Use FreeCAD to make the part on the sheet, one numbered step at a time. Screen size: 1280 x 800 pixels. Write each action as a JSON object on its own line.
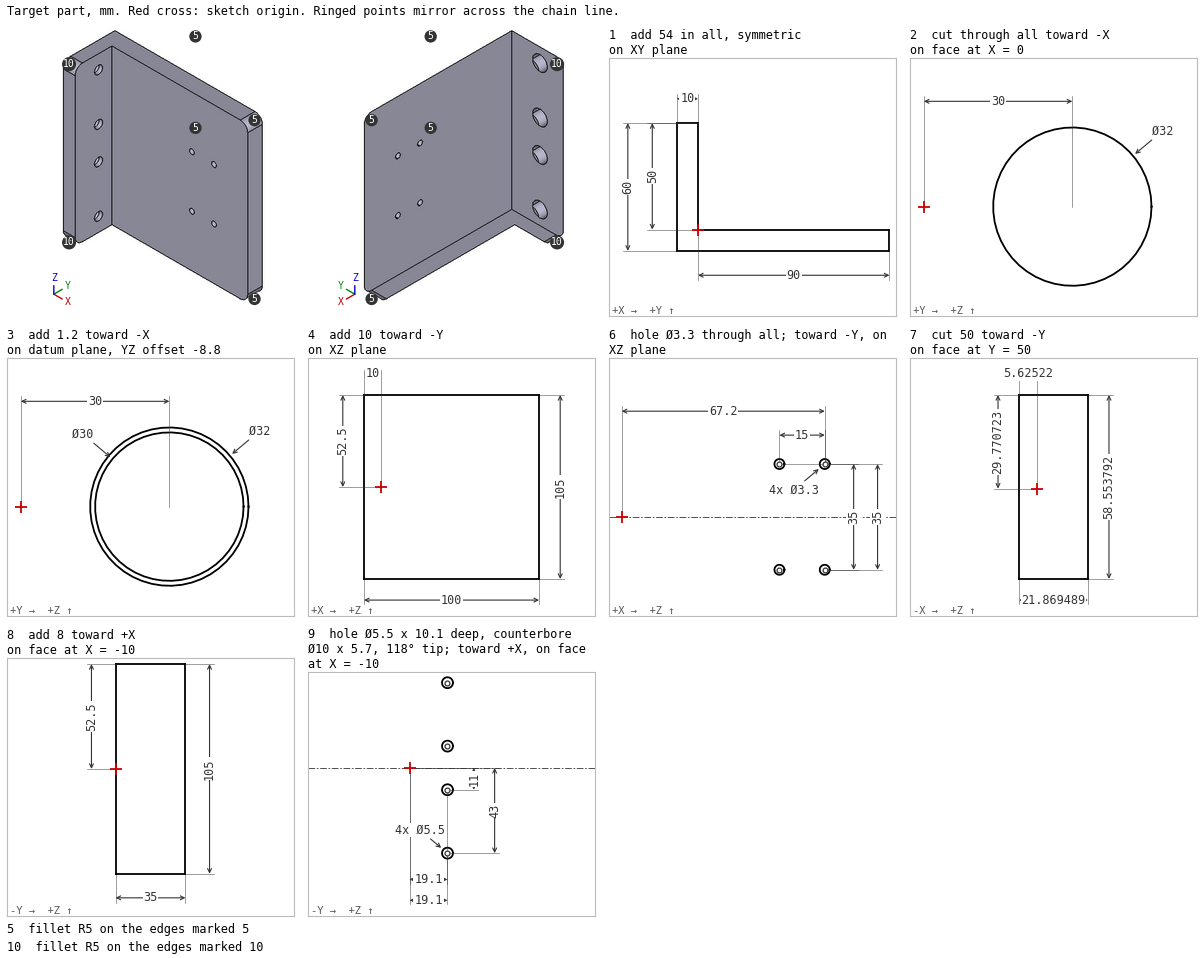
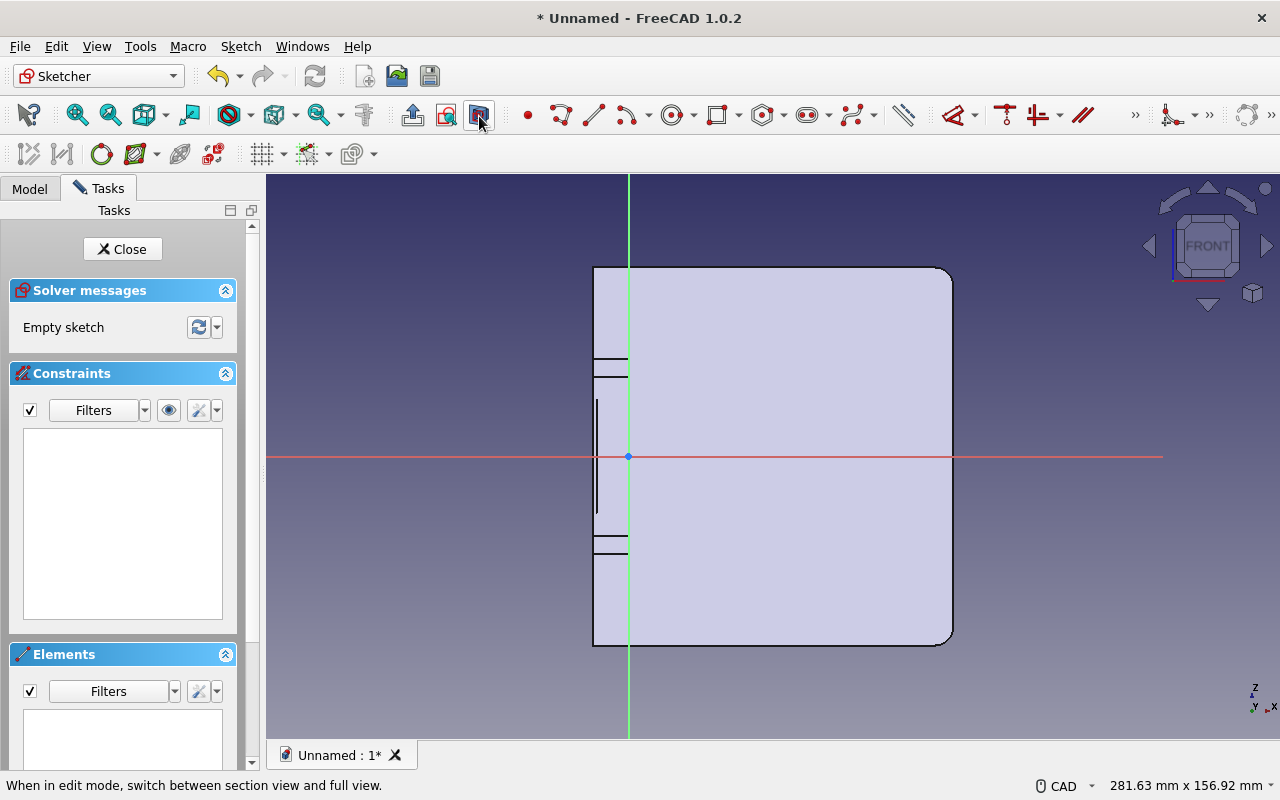
{"action": "scroll", "coordinate": [792, 456], "scroll_direction": "up", "scroll_amount": 4}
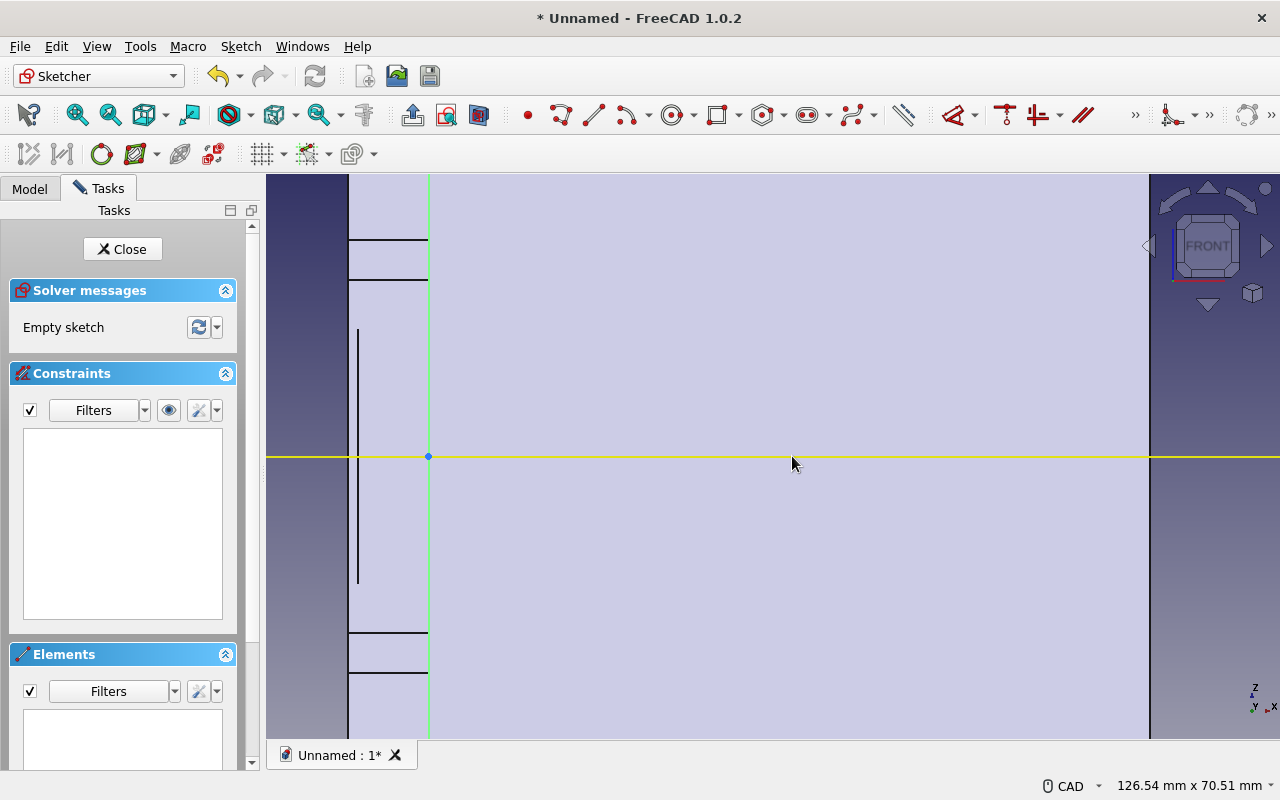
{"action": "left_click", "coordinate": [672, 116]}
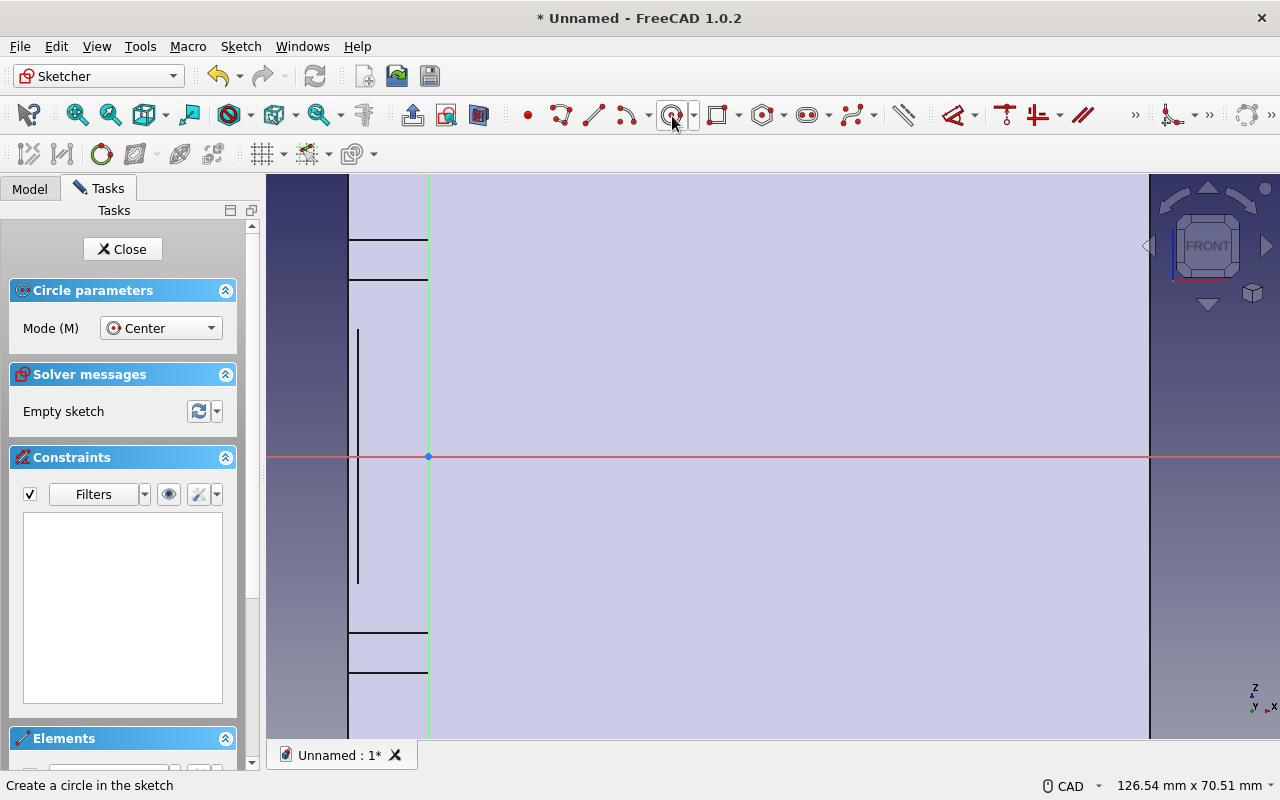
{"action": "scroll", "coordinate": [967, 316], "scroll_direction": "up", "scroll_amount": 3}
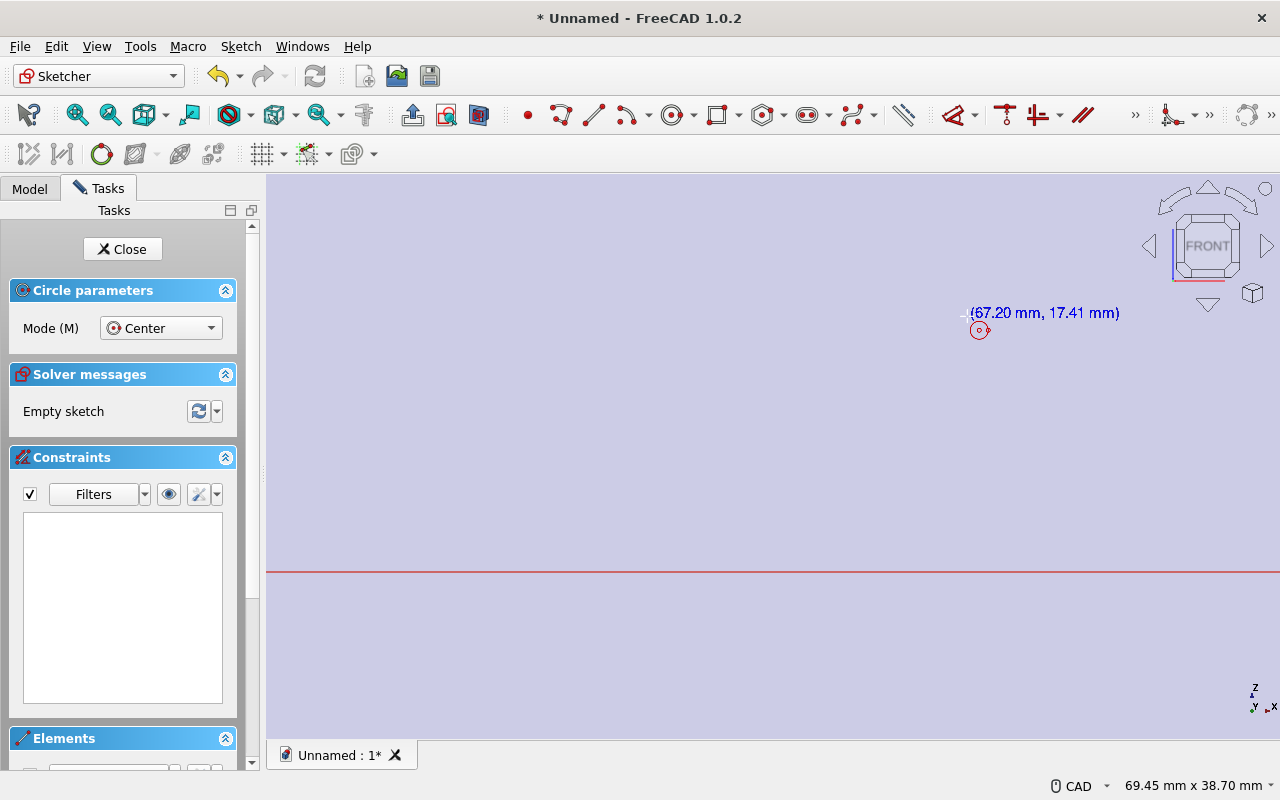
{"action": "left_click", "coordinate": [966, 316]}
{"action": "mouse_move", "coordinate": [984, 299]}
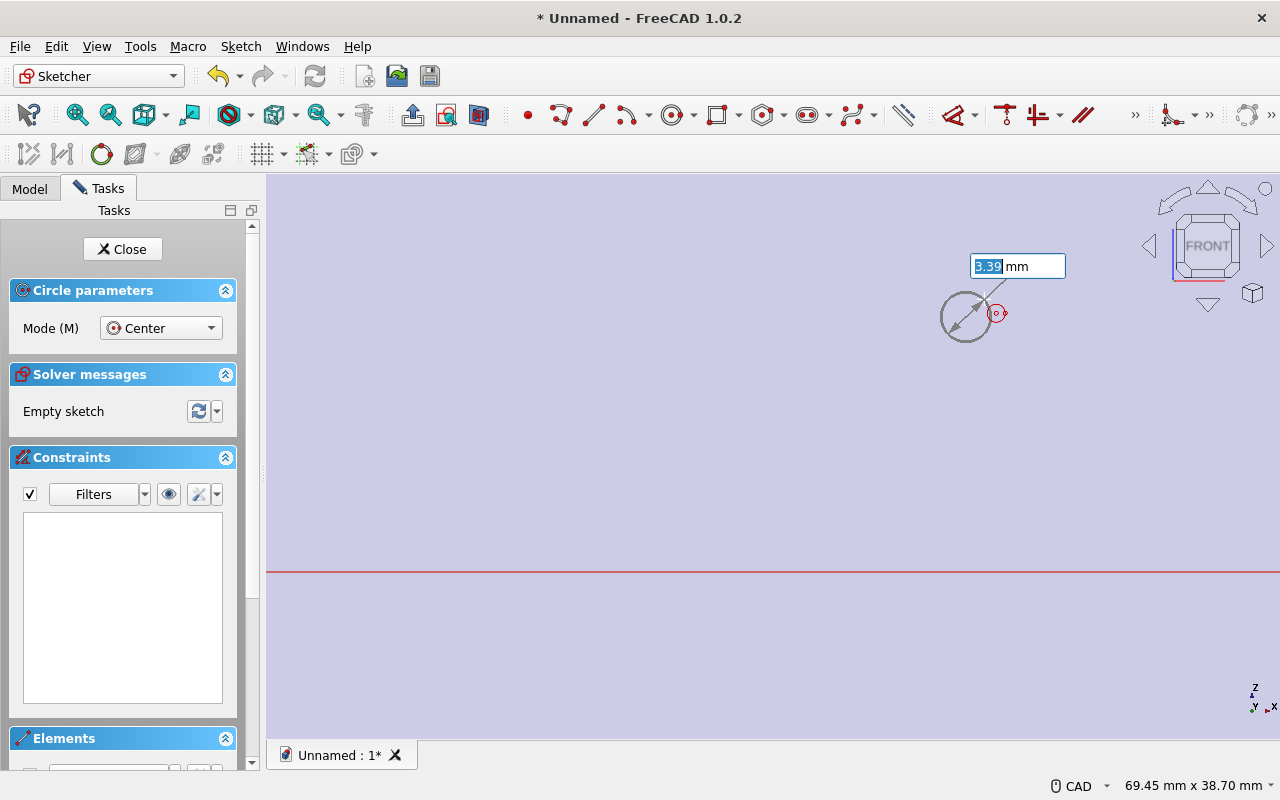
{"action": "type", "text": "3.3"}
{"action": "key", "text": "Return"}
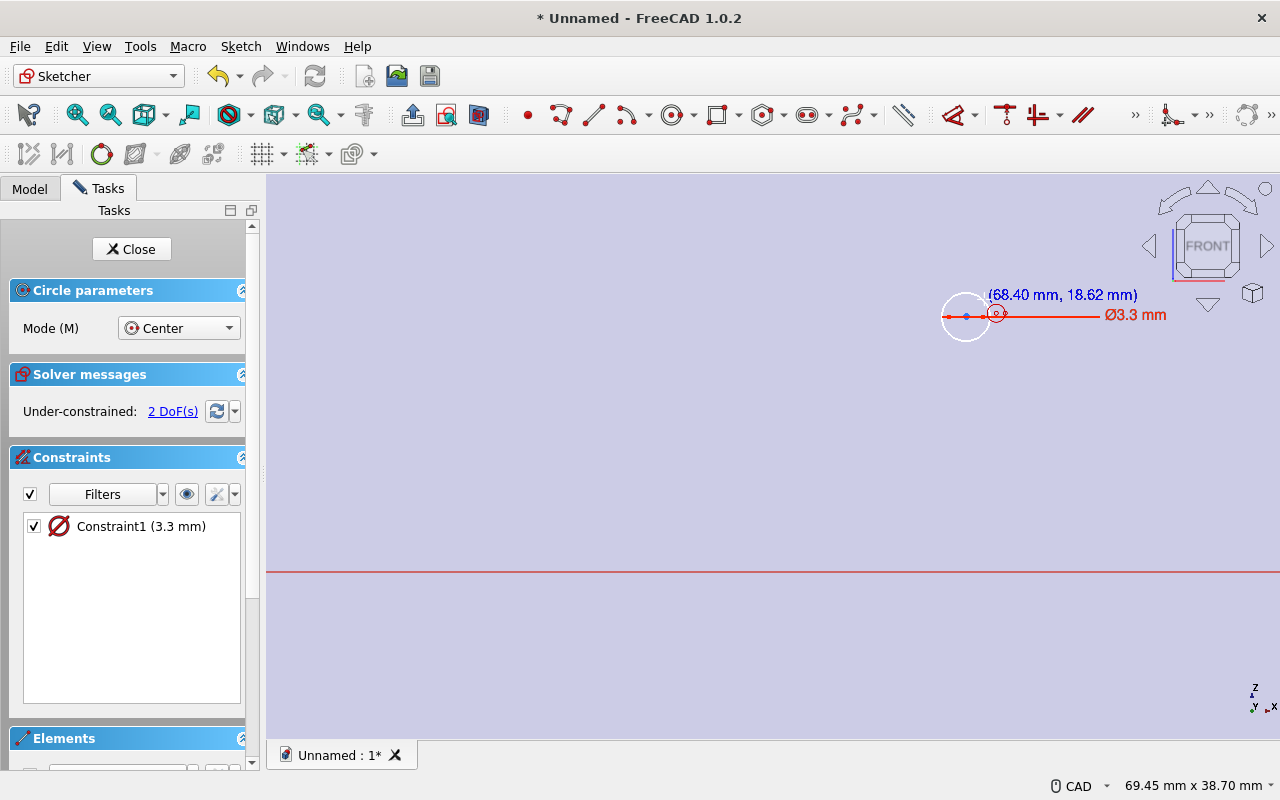
{"action": "left_click", "coordinate": [747, 316]}
{"action": "mouse_move", "coordinate": [765, 299]}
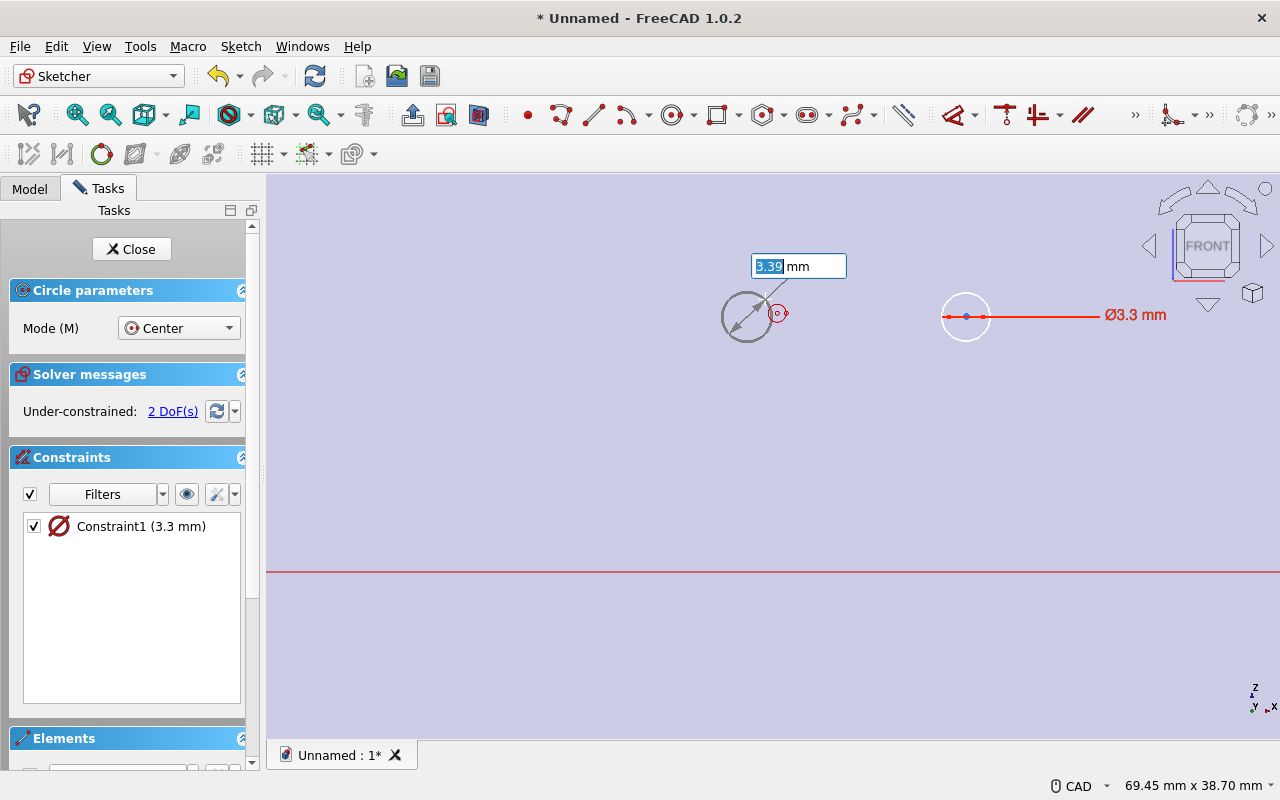
{"action": "type", "text": "3.3"}
{"action": "key", "text": "Return"}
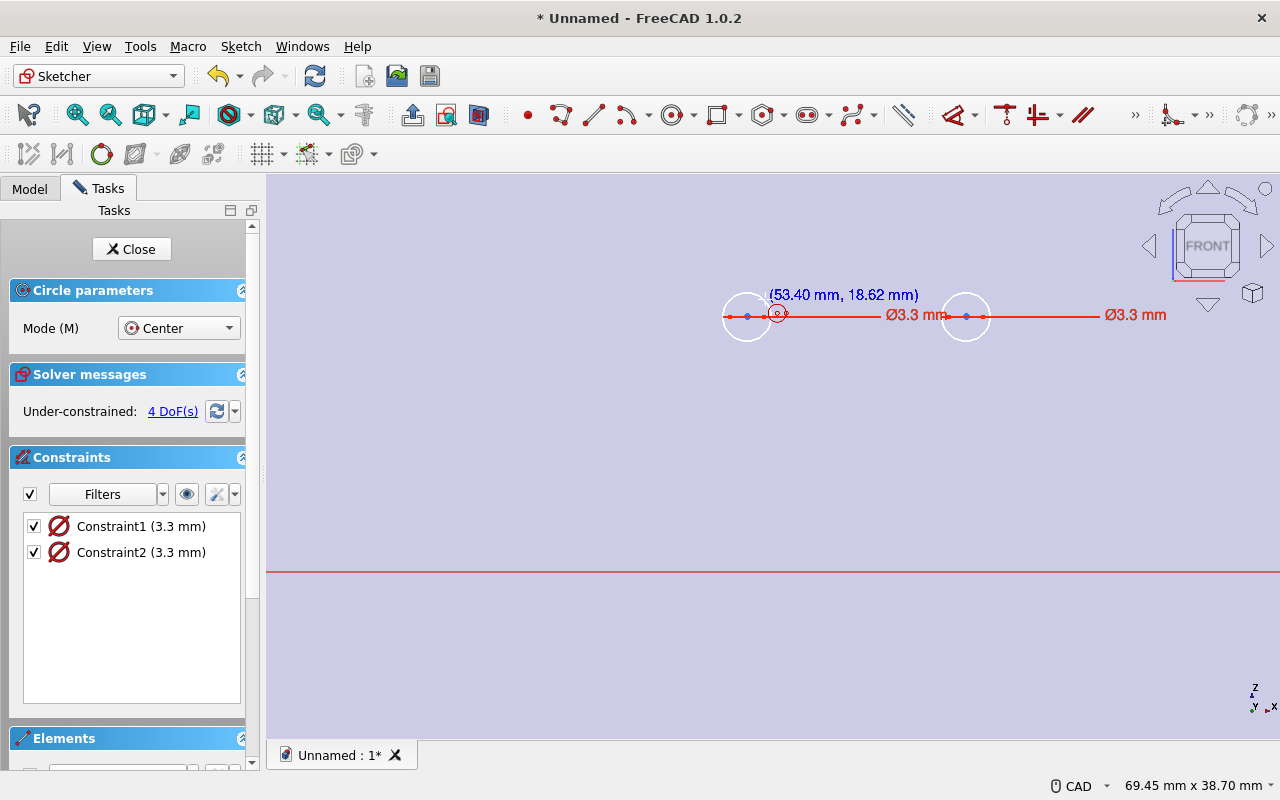
{"action": "scroll", "coordinate": [968, 316], "scroll_direction": "down", "scroll_amount": 3}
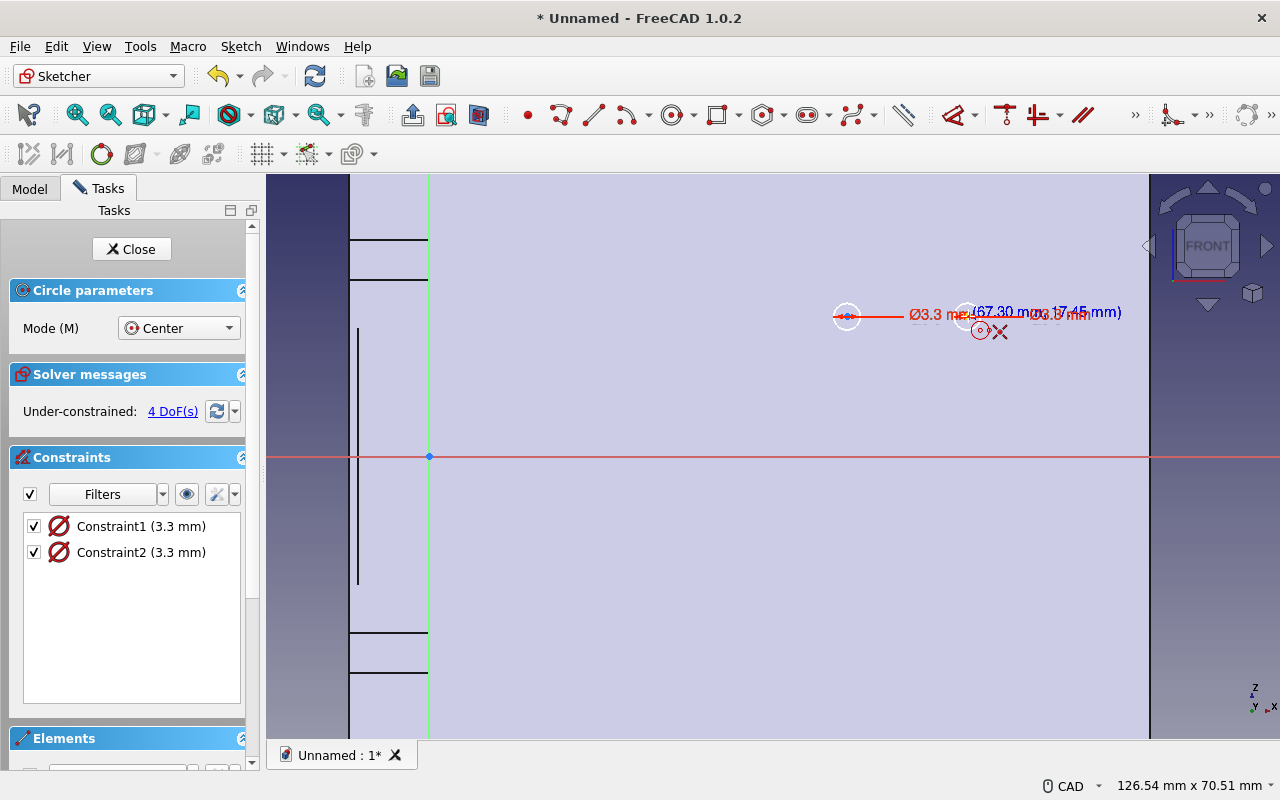
{"action": "scroll", "coordinate": [967, 597], "scroll_direction": "up", "scroll_amount": 3}